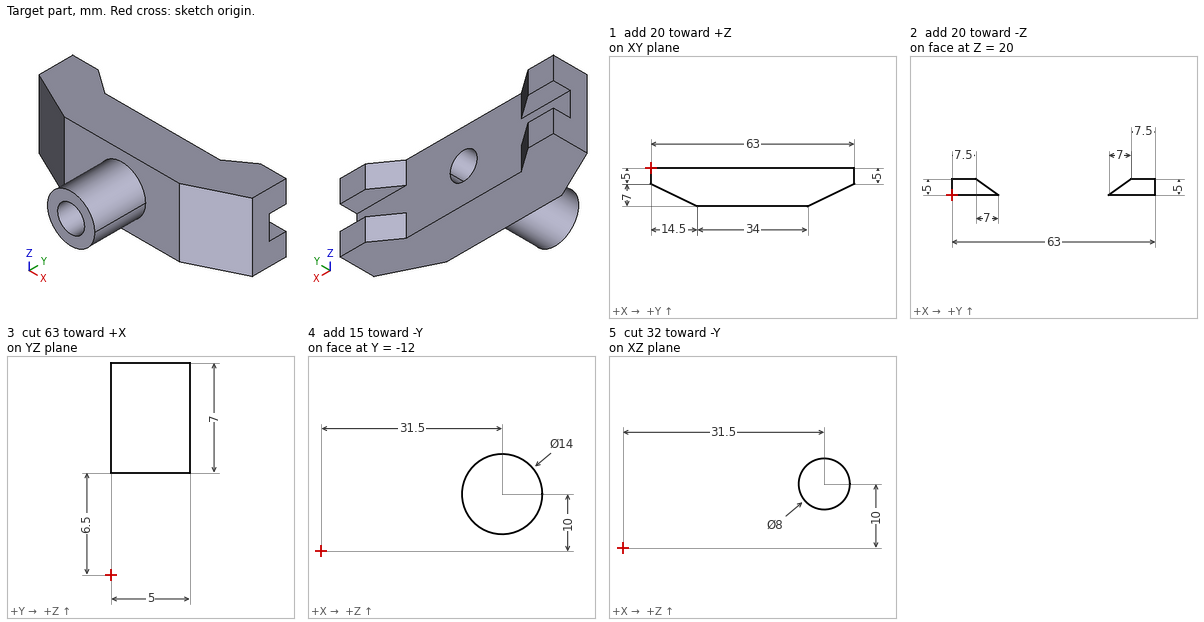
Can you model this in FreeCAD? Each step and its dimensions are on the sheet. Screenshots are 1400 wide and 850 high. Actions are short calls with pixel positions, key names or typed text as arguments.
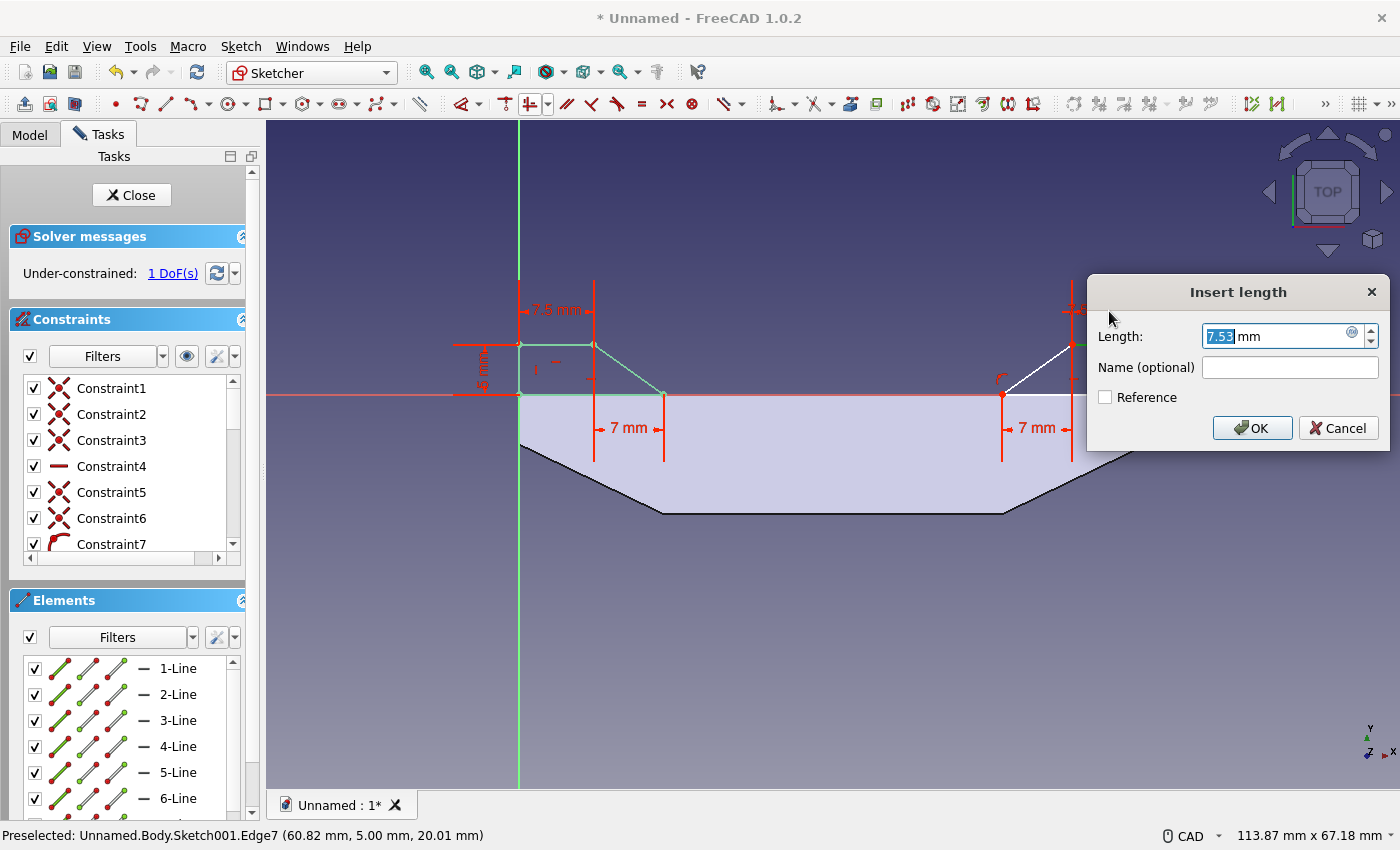
text(7.5)
key(Return)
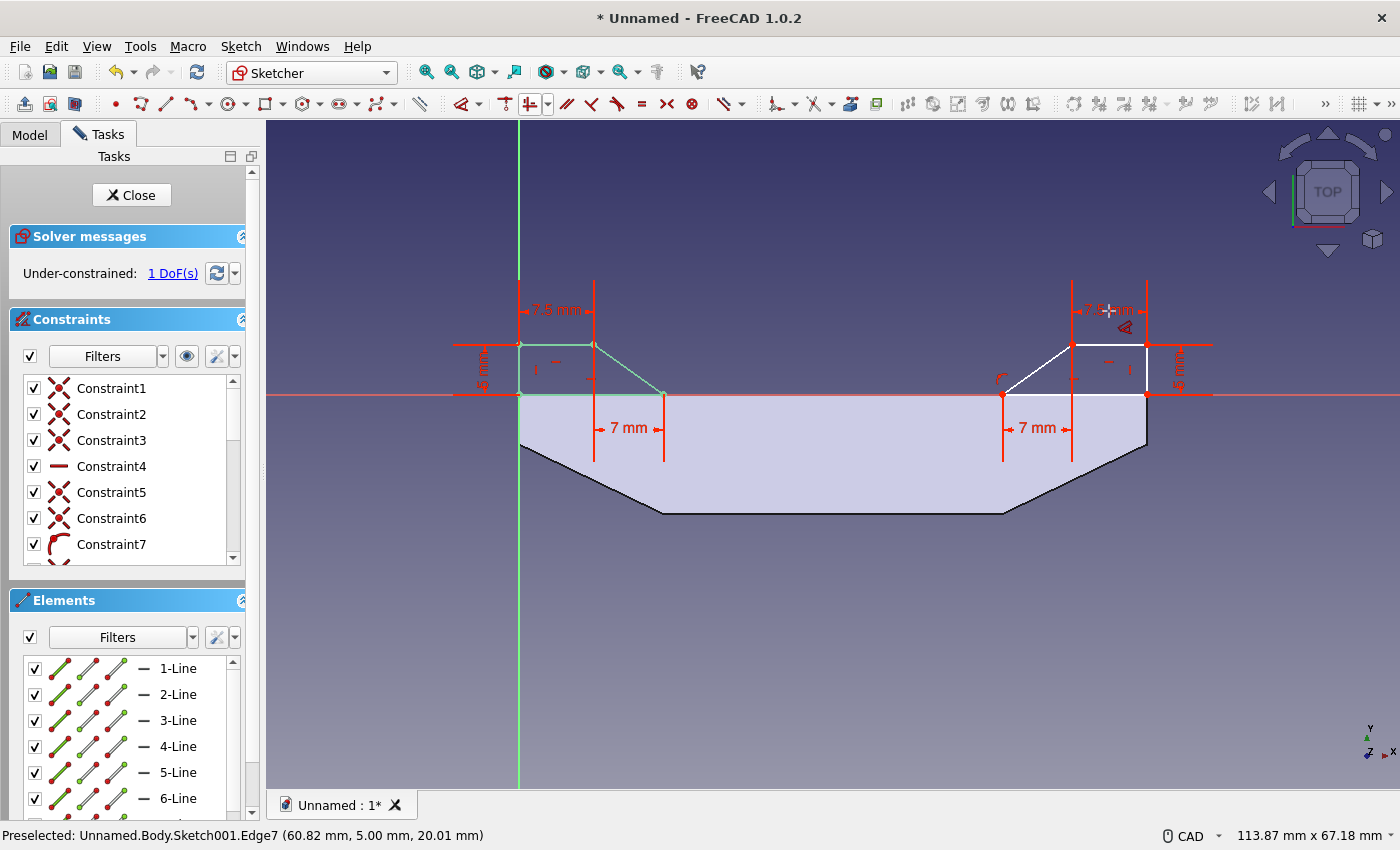
click(1147, 395)
click(833, 429)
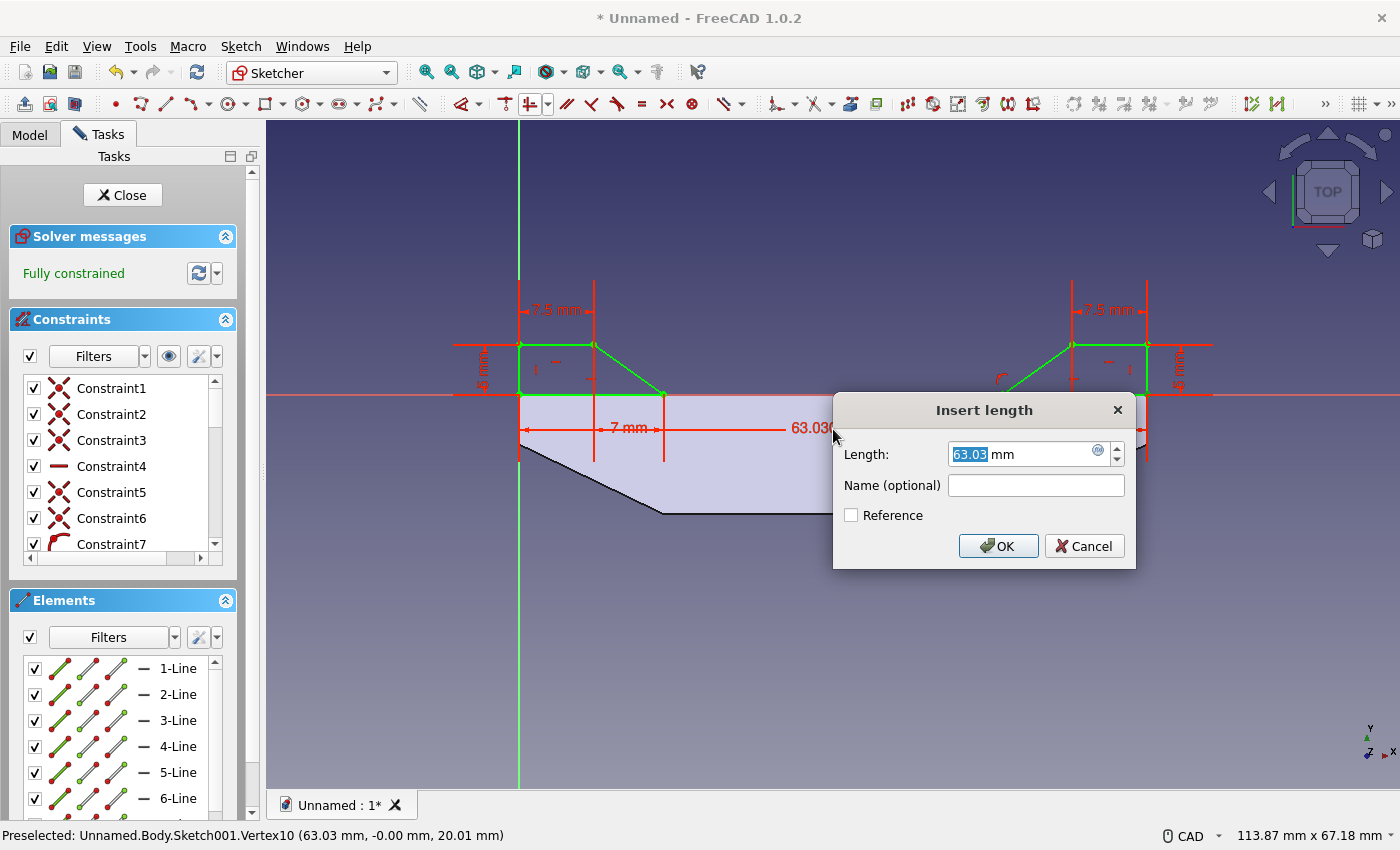
text(63)
key(Return)
key(Escape)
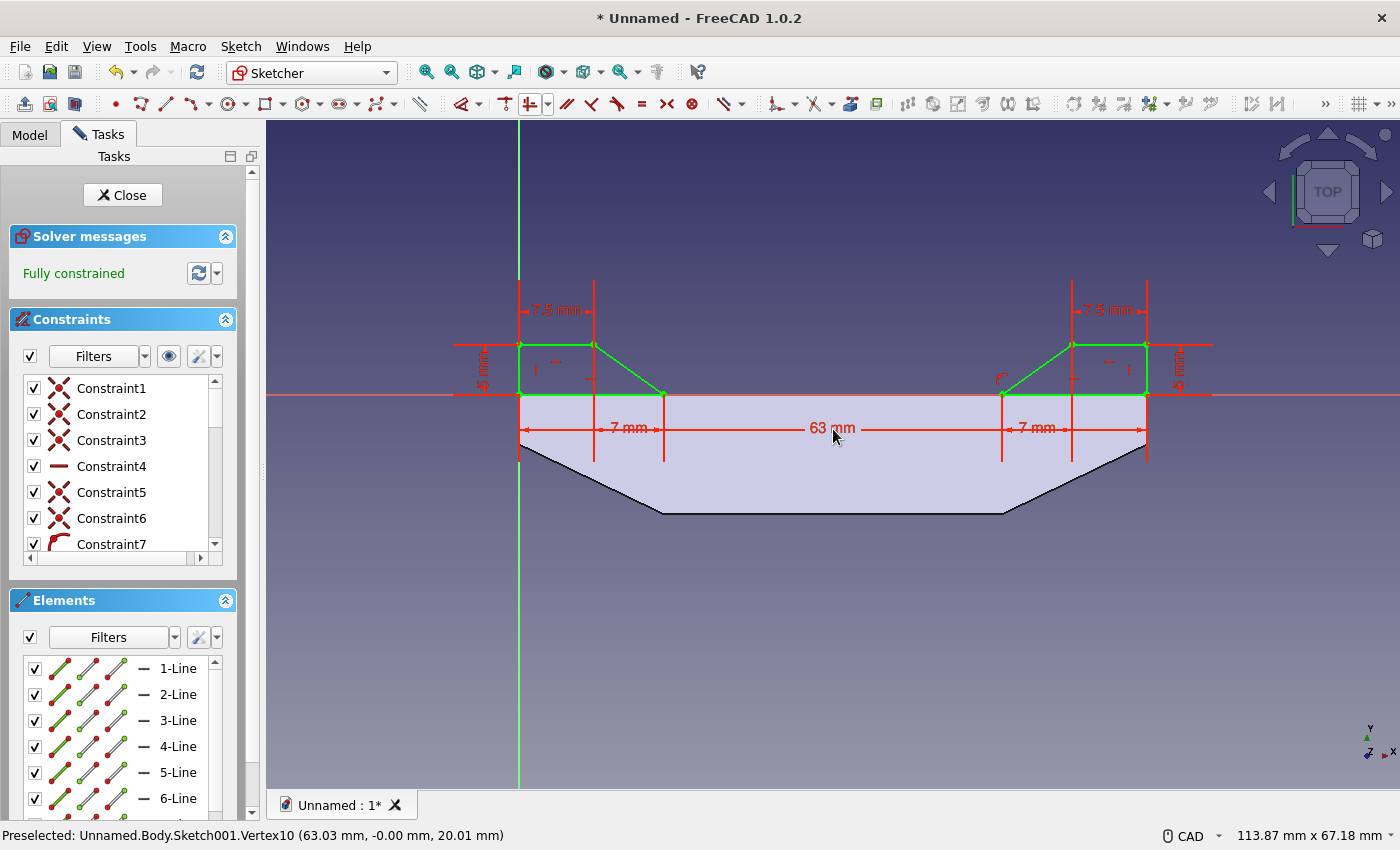
click(123, 195)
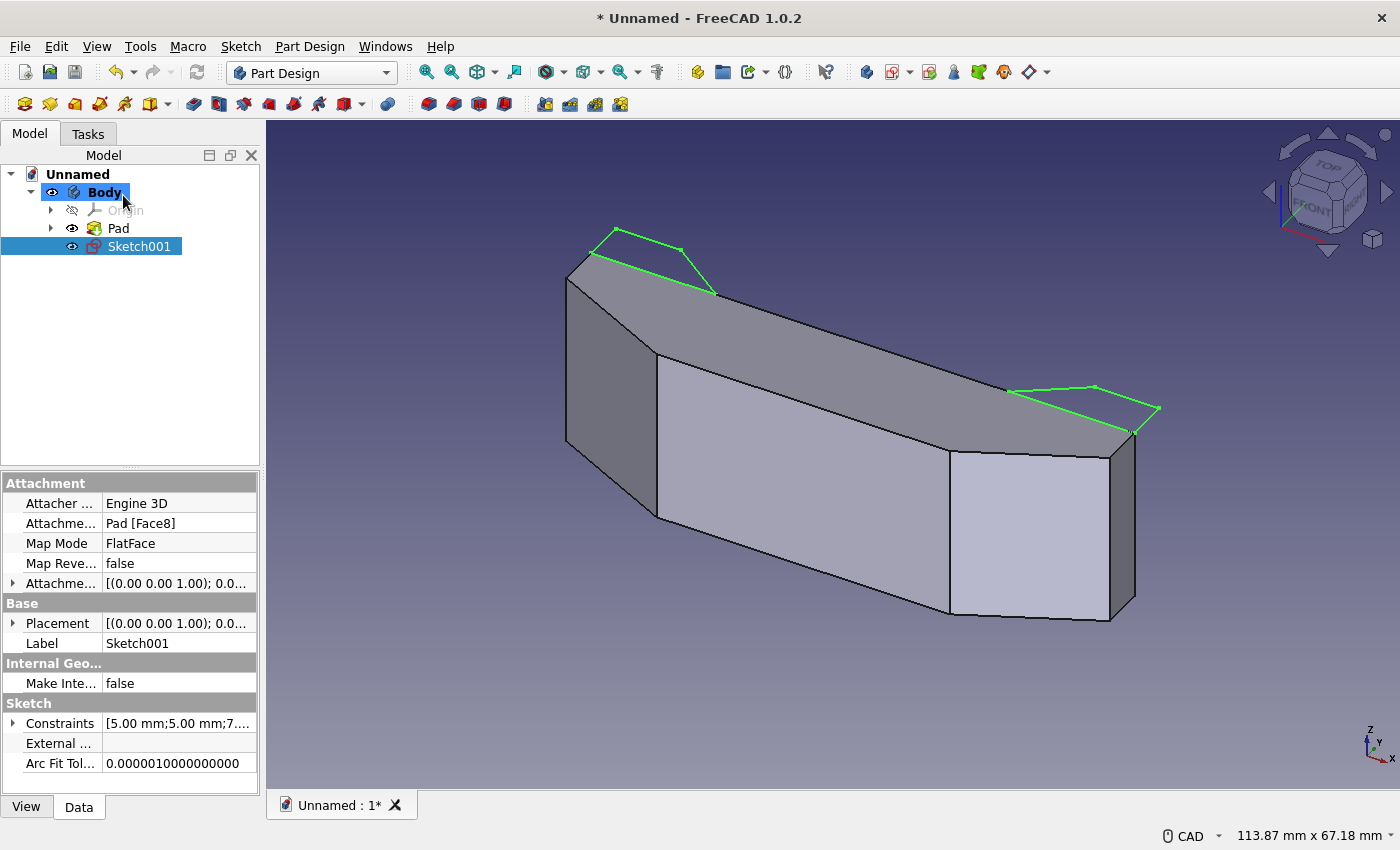
click(25, 104)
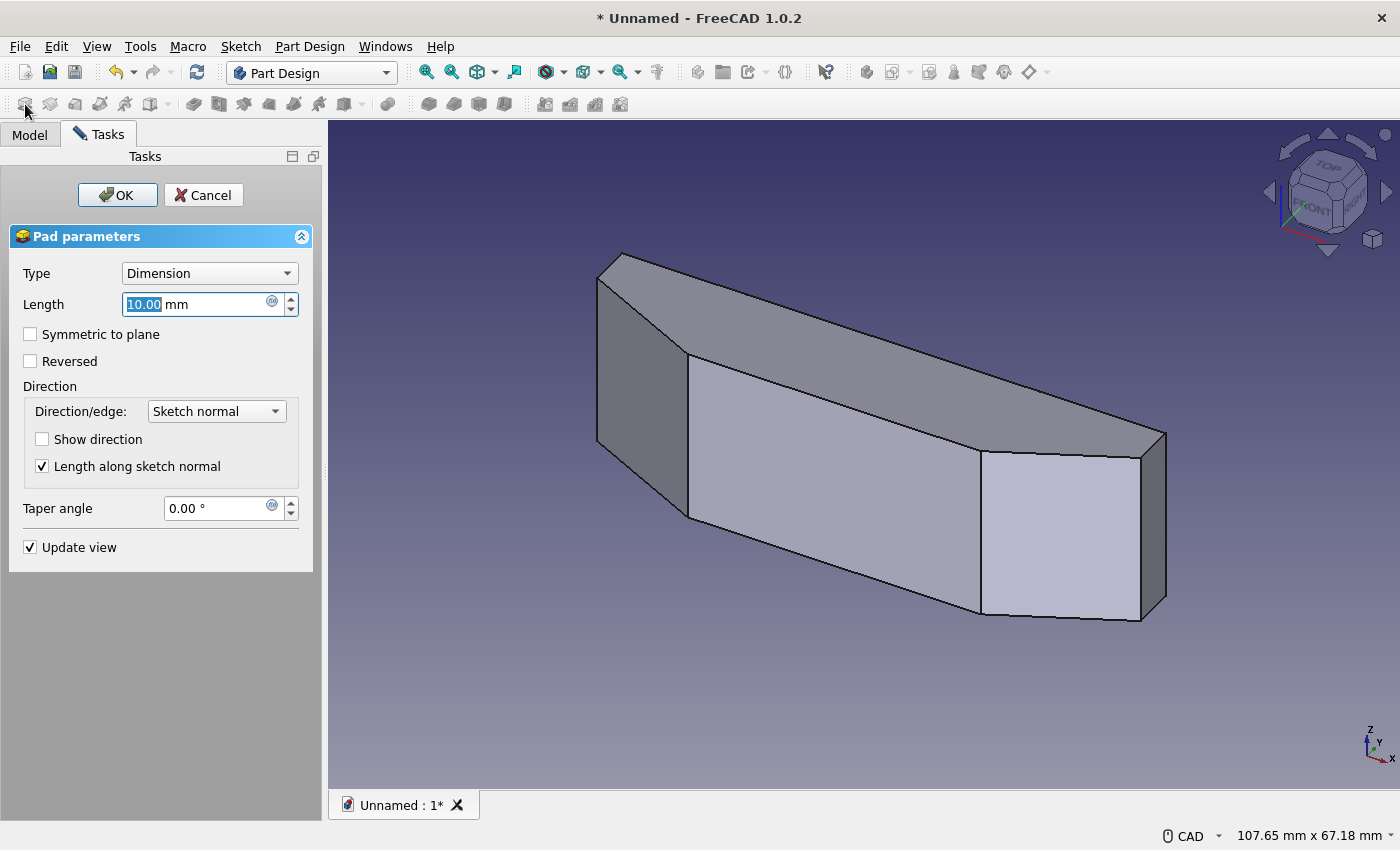
text(20)
key(Tab)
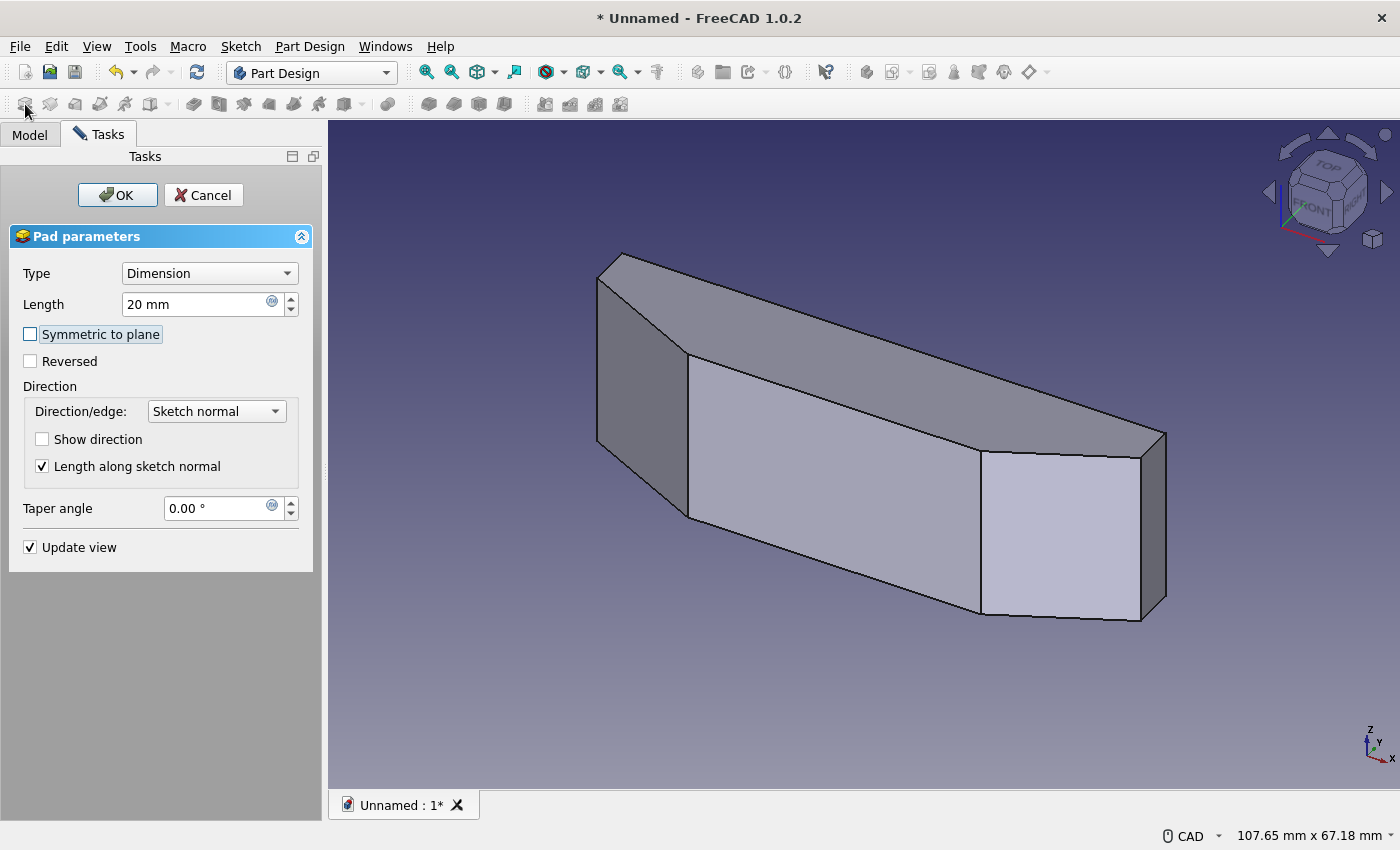
click(31, 361)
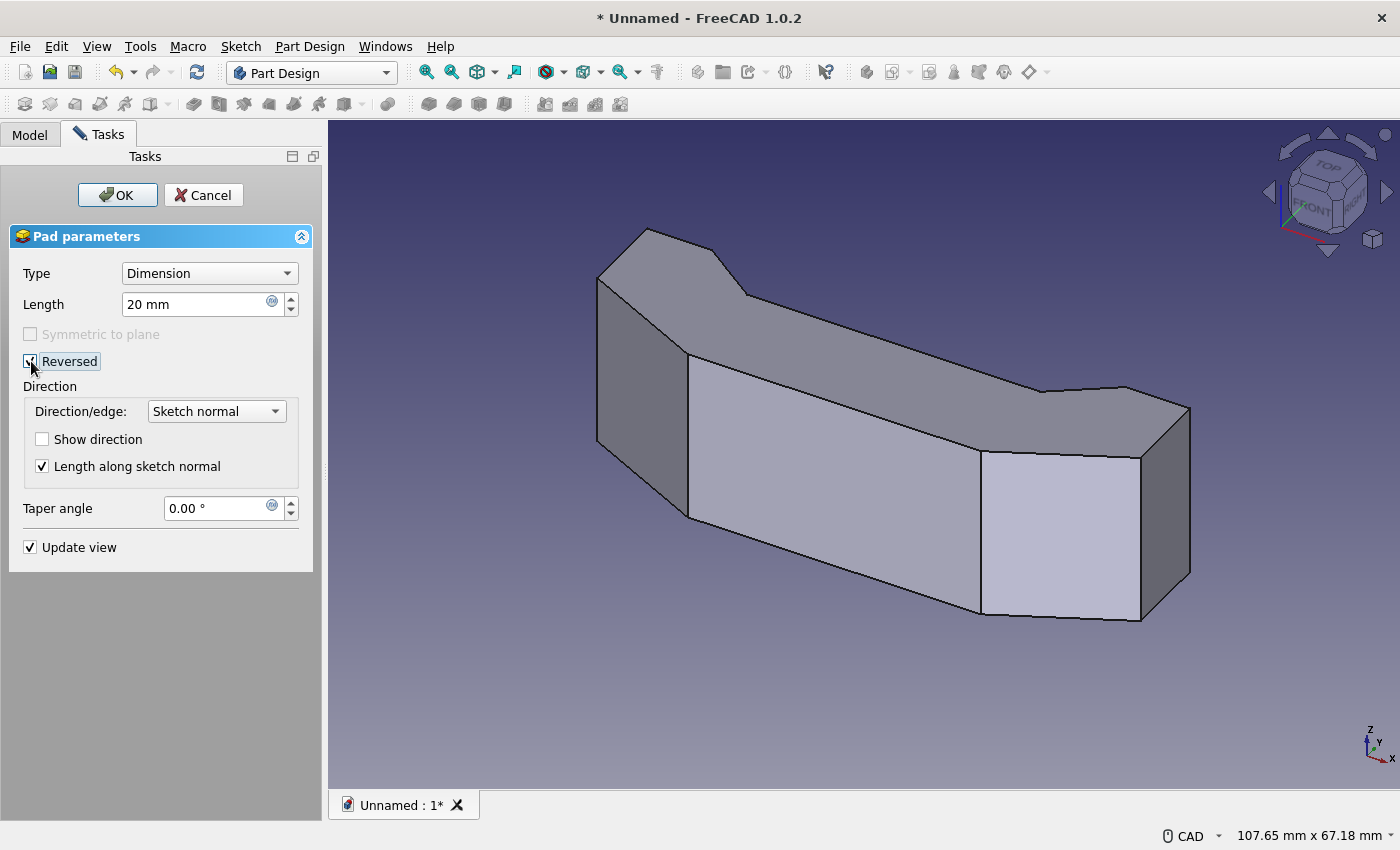
click(118, 195)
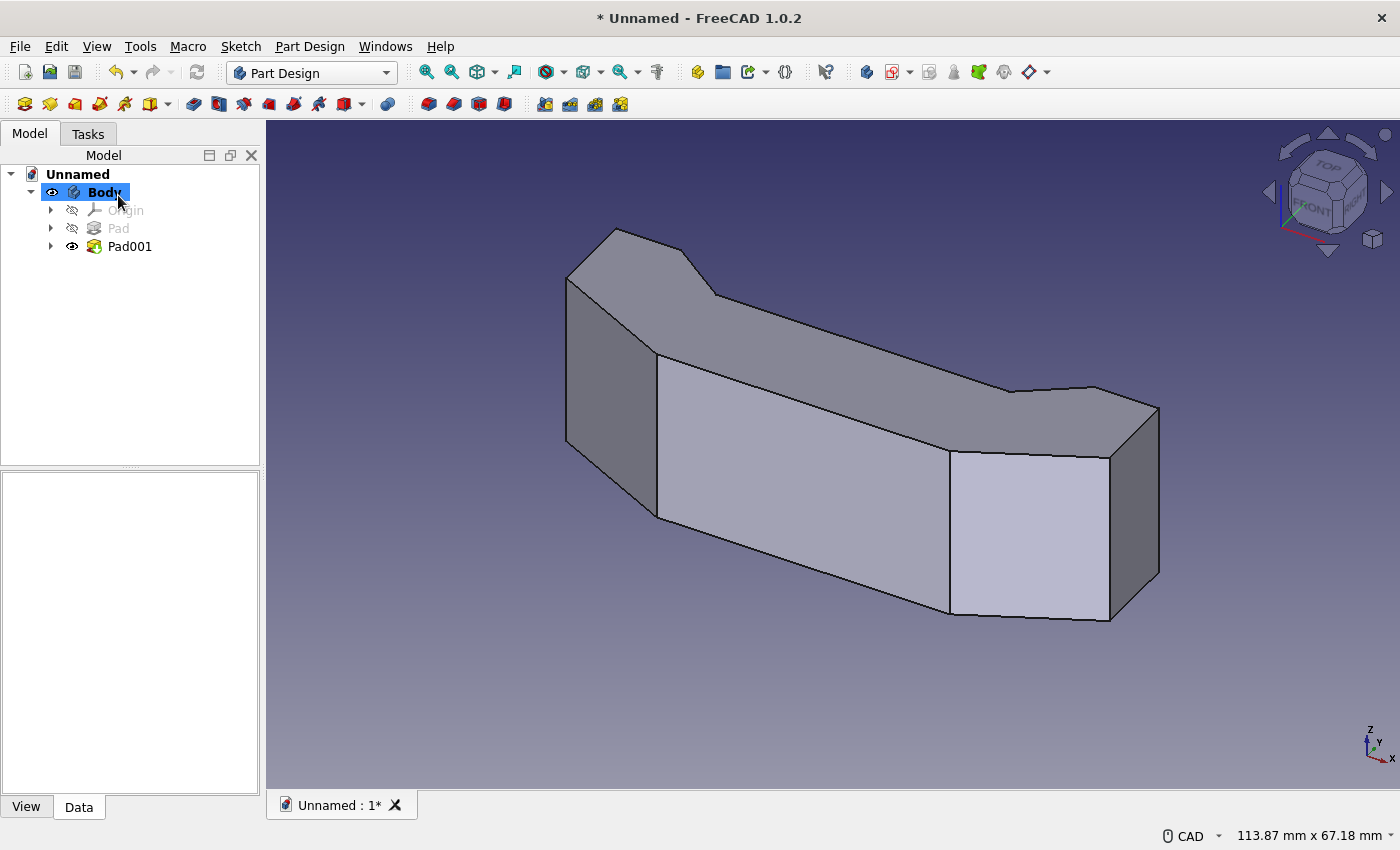
click(892, 72)